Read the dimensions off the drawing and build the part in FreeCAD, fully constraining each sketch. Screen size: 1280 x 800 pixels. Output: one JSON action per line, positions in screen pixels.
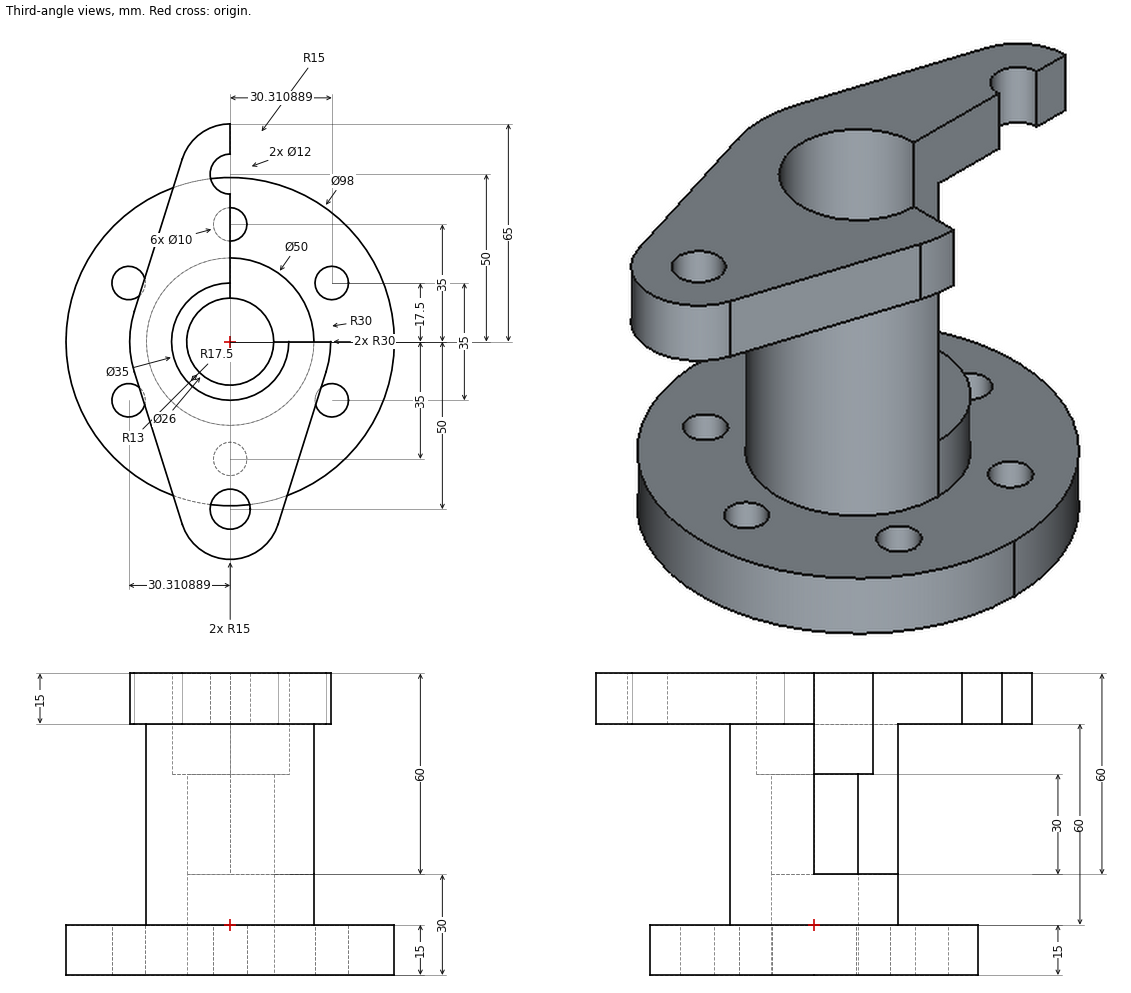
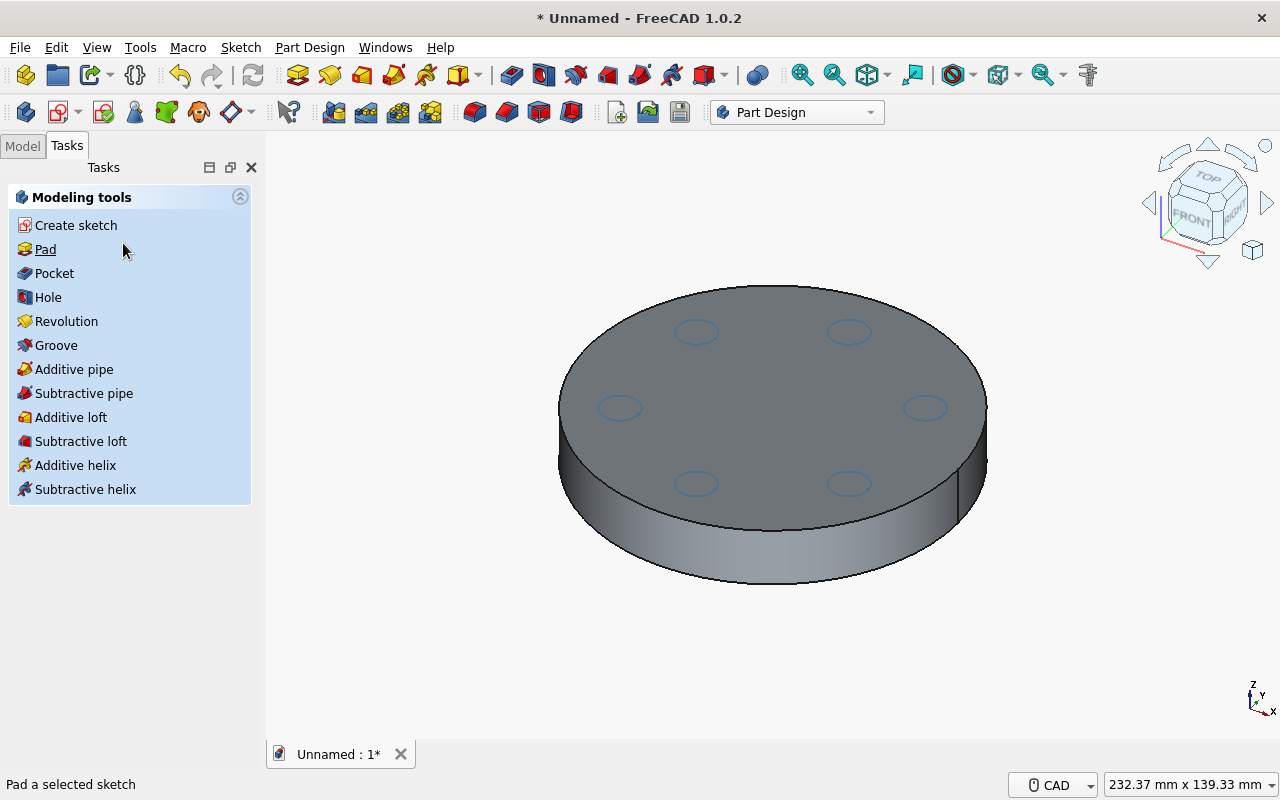
{"action": "left_click", "coordinate": [512, 76]}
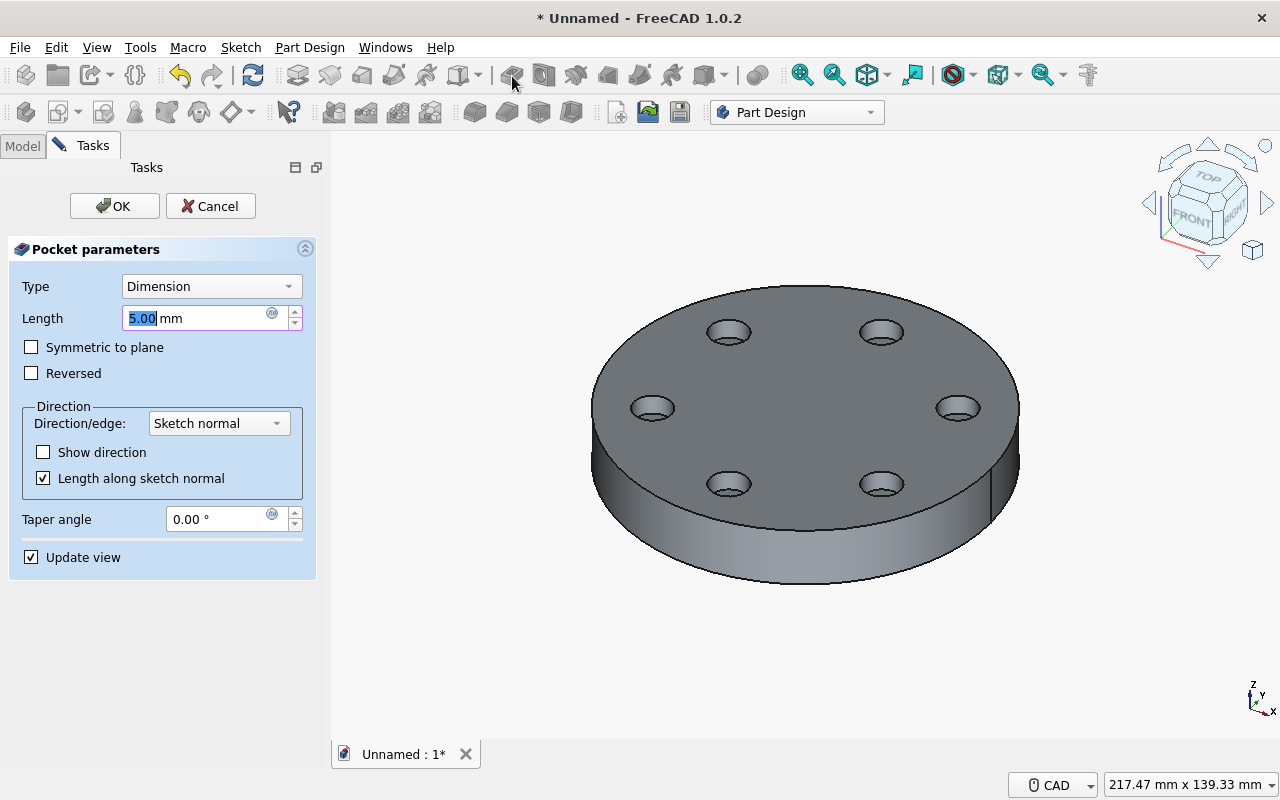
{"action": "type", "text": "15"}
{"action": "key", "text": "Tab"}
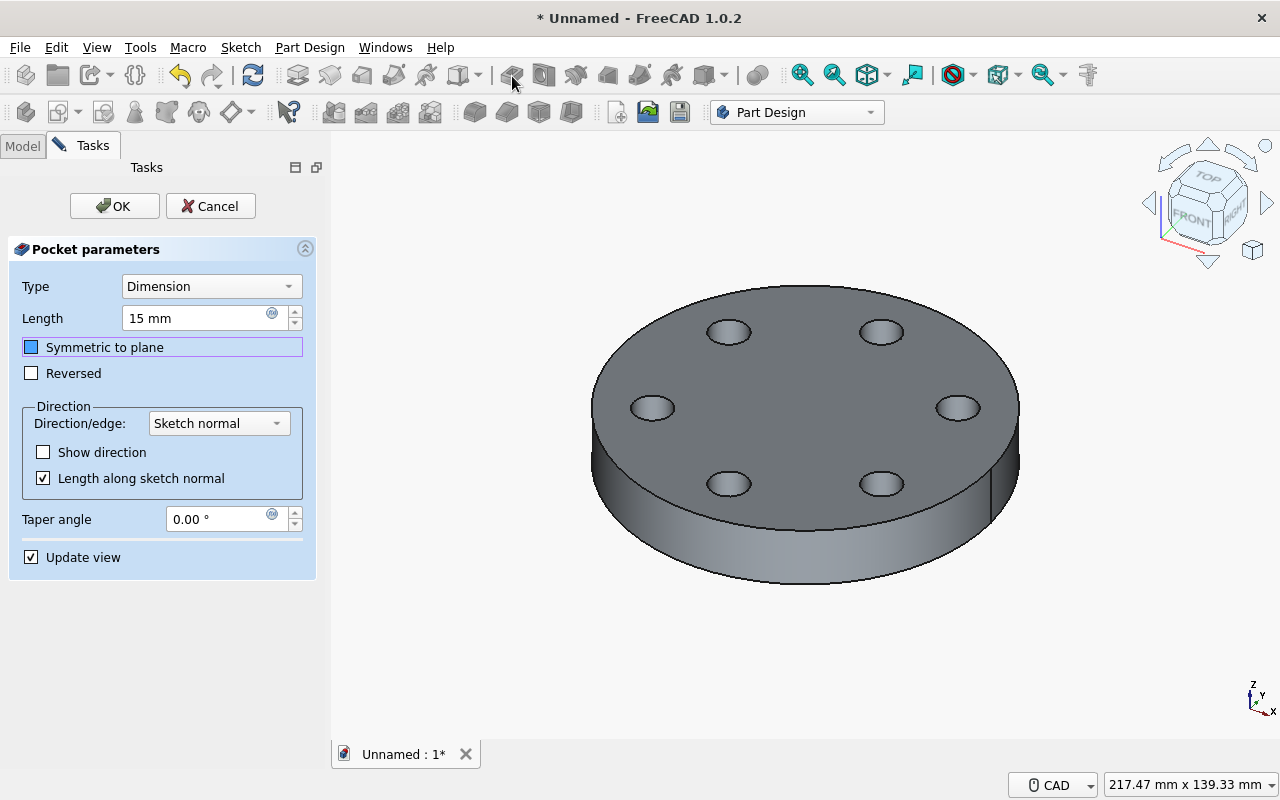
{"action": "left_click", "coordinate": [115, 206]}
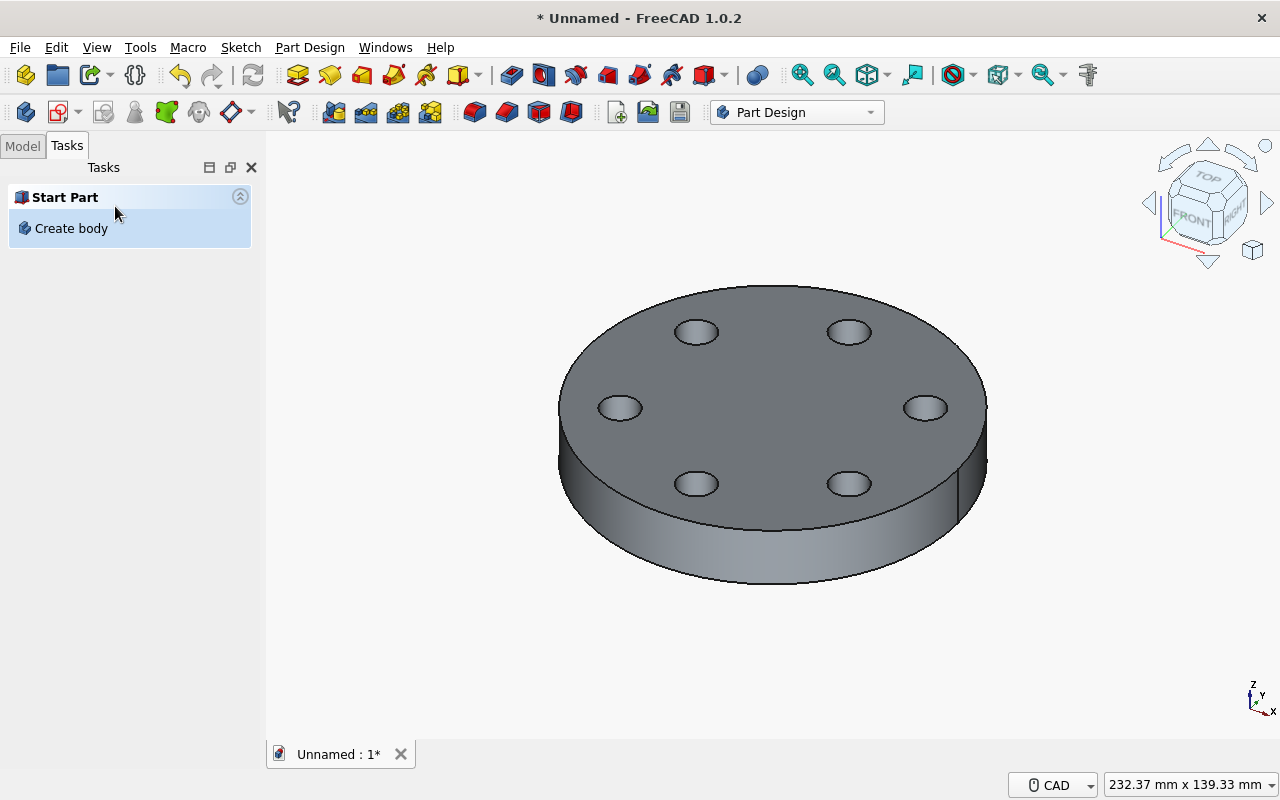
{"action": "left_click", "coordinate": [773, 407]}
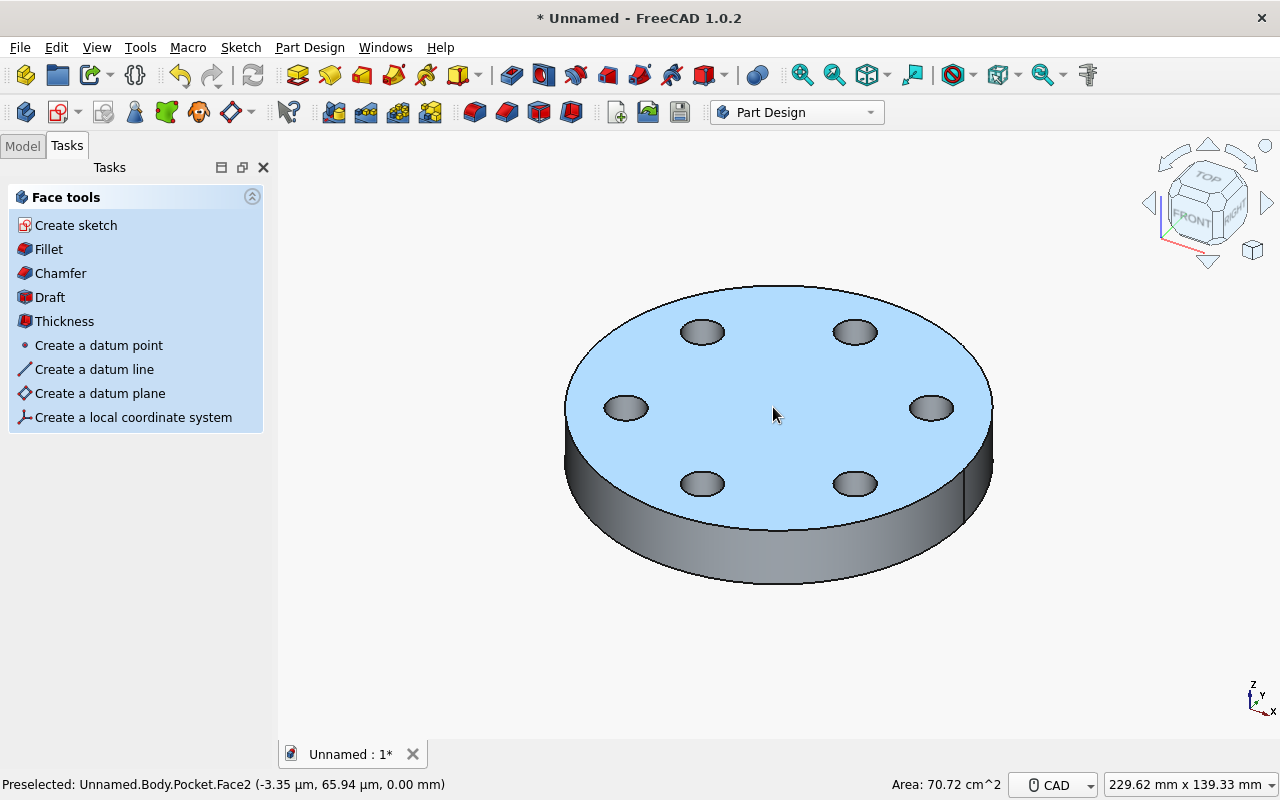
{"action": "left_click", "coordinate": [58, 112]}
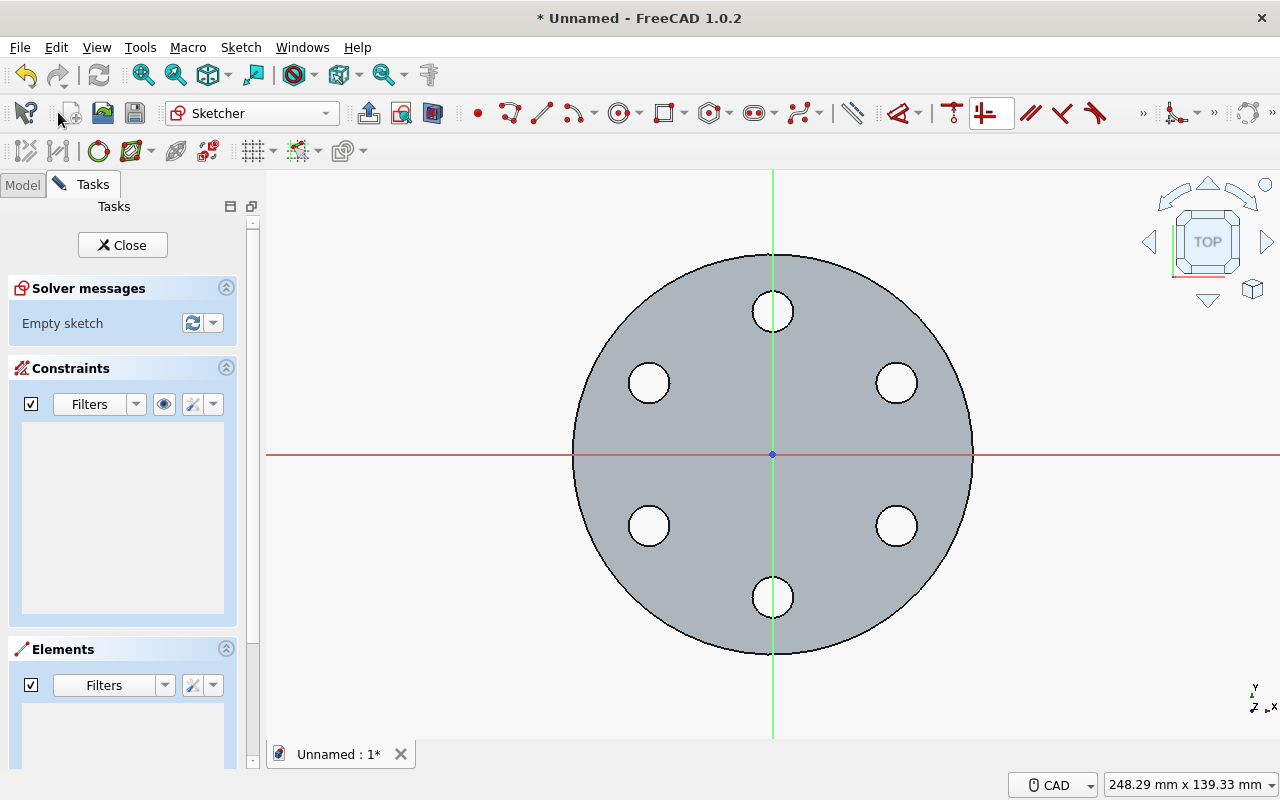
{"action": "scroll", "coordinate": [856, 454], "scroll_direction": "up", "scroll_amount": 3}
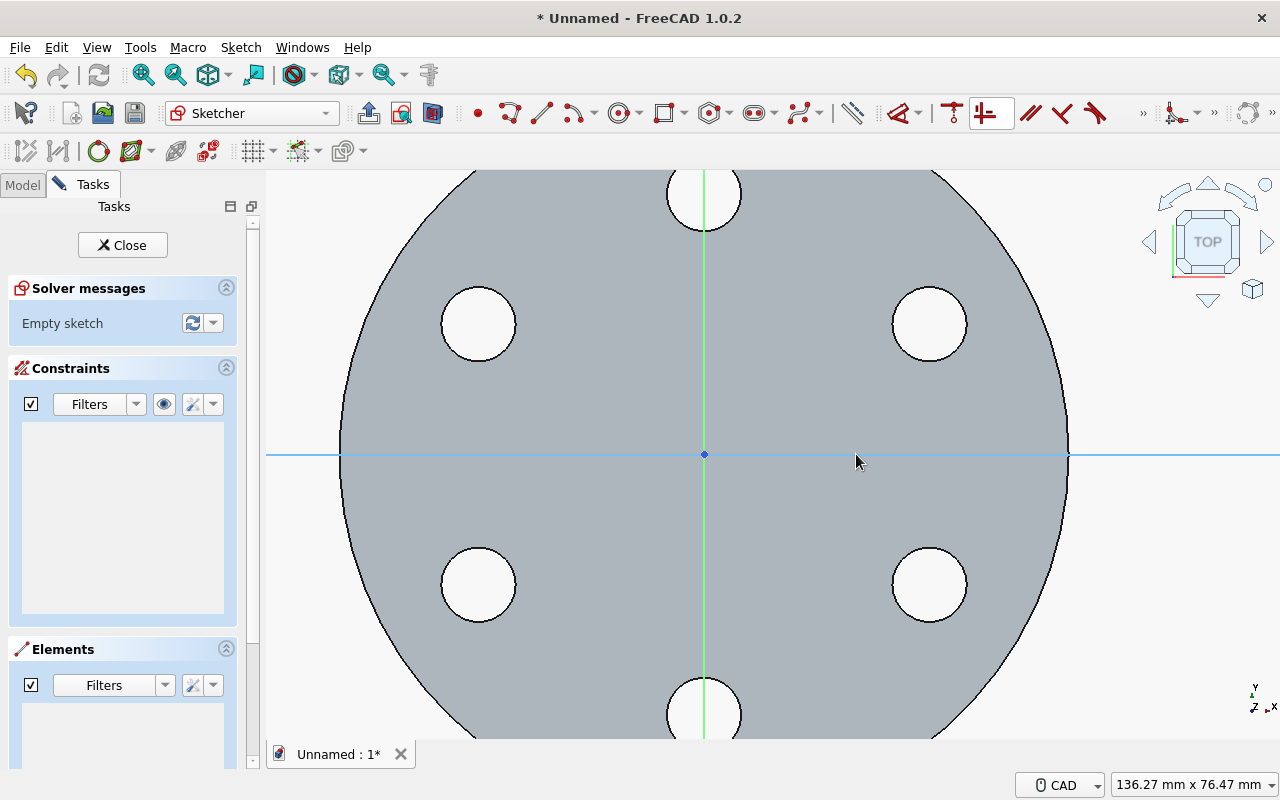
{"action": "left_click", "coordinate": [620, 114]}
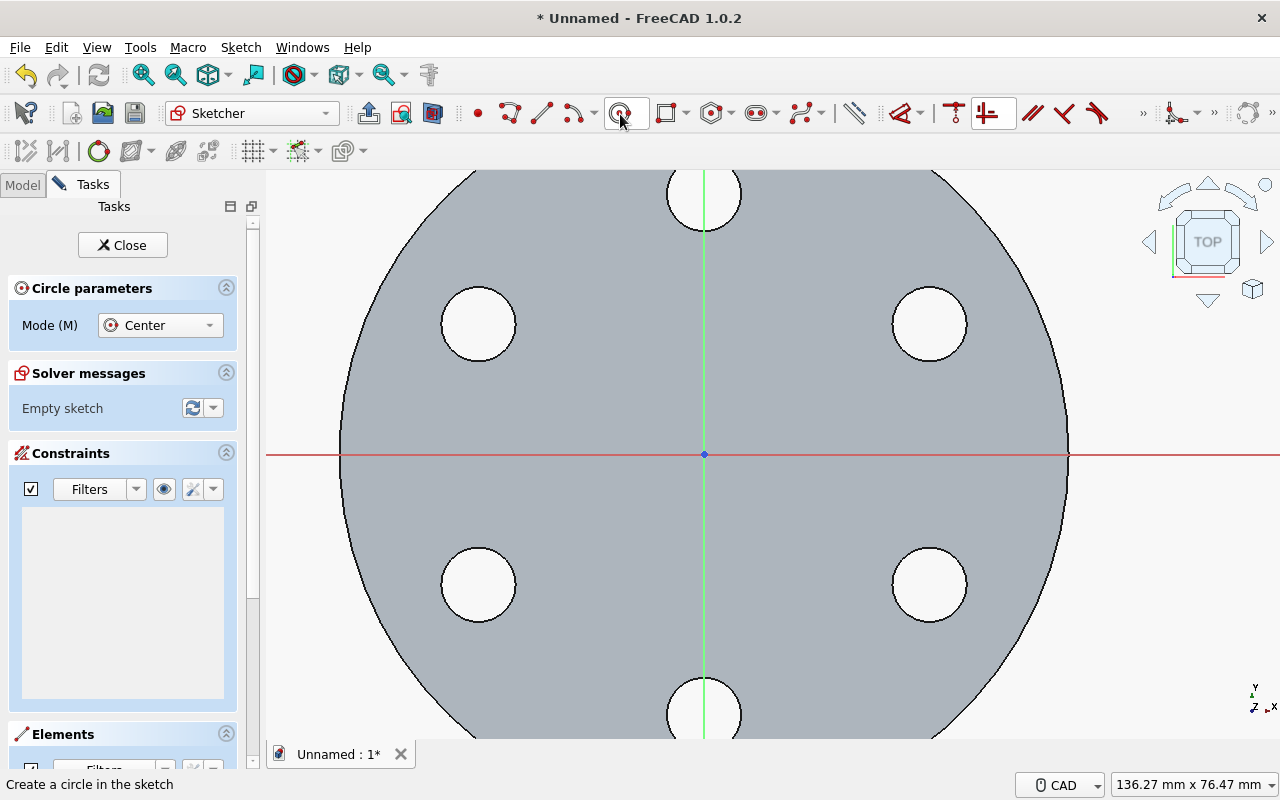
{"action": "left_click", "coordinate": [704, 454]}
{"action": "left_click", "coordinate": [836, 323]}
{"action": "key", "text": "Escape"}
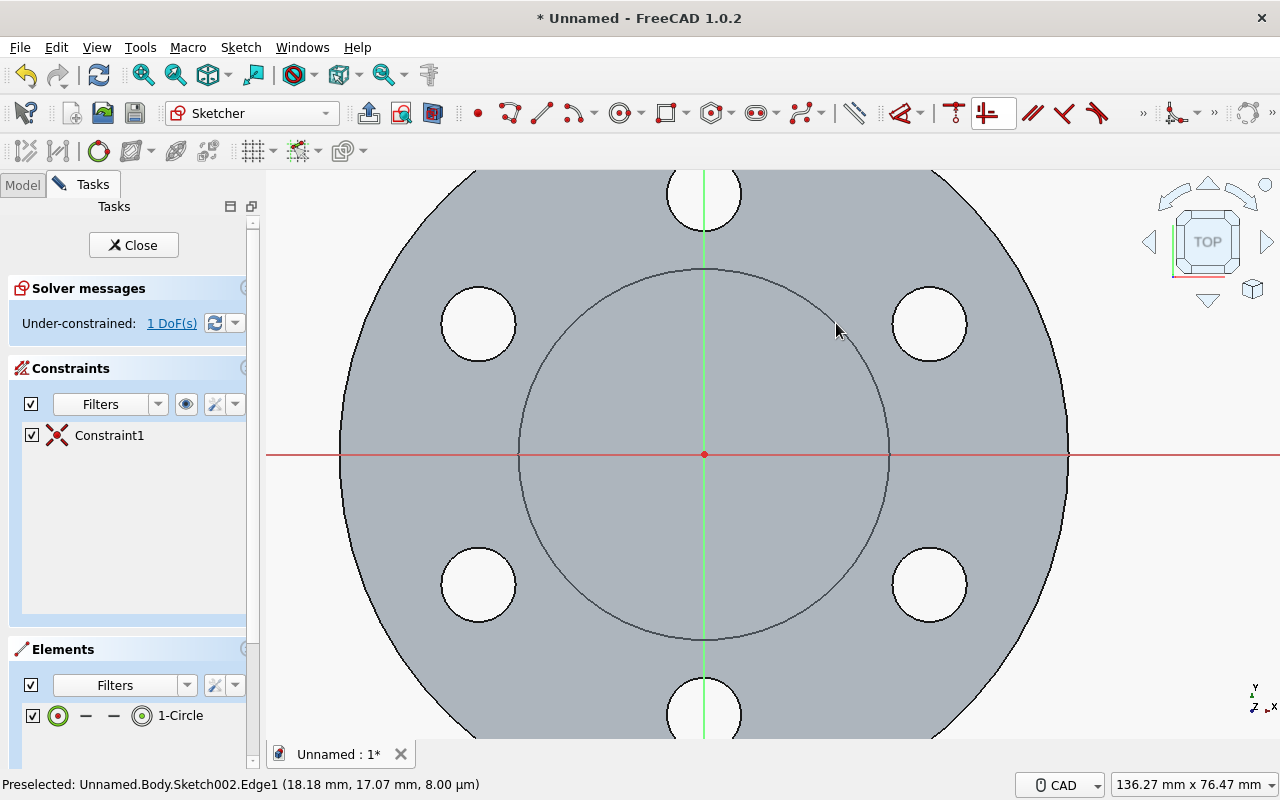
{"action": "left_click", "coordinate": [835, 323]}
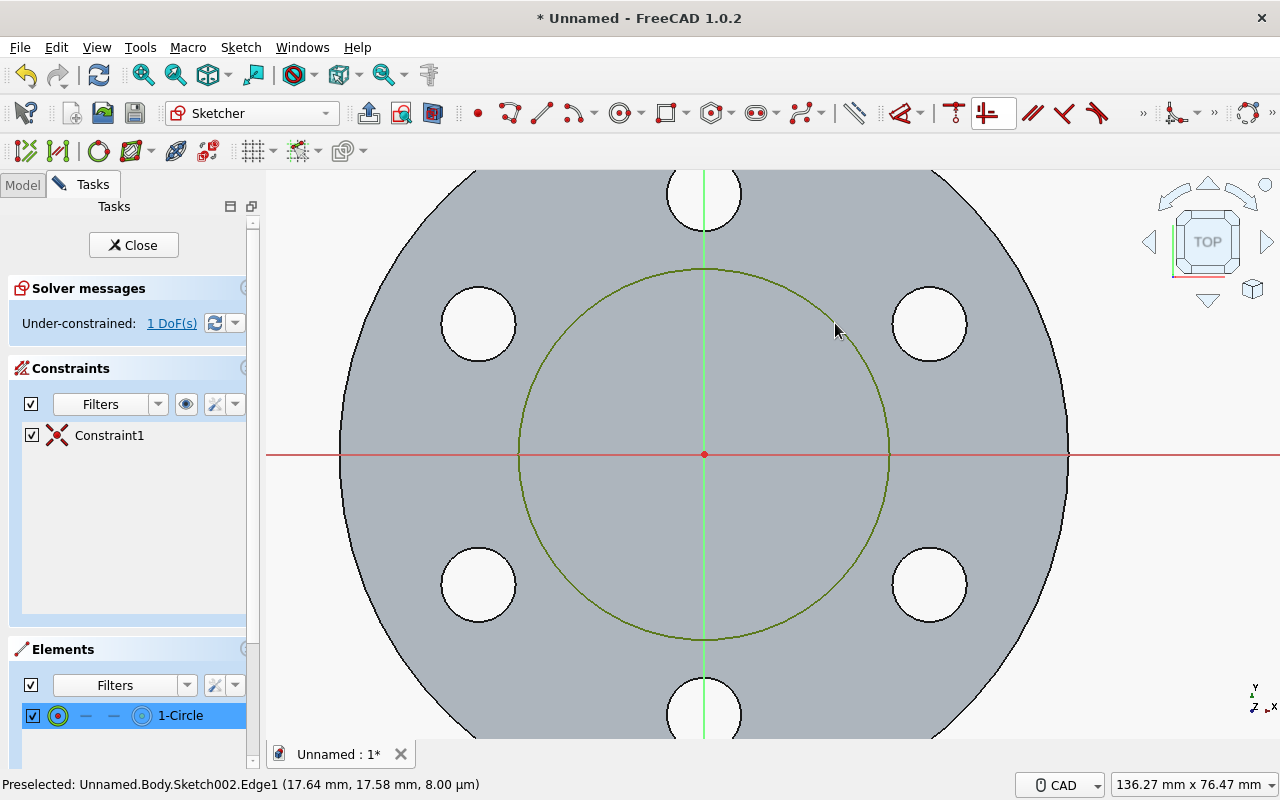
{"action": "left_click", "coordinate": [922, 114]}